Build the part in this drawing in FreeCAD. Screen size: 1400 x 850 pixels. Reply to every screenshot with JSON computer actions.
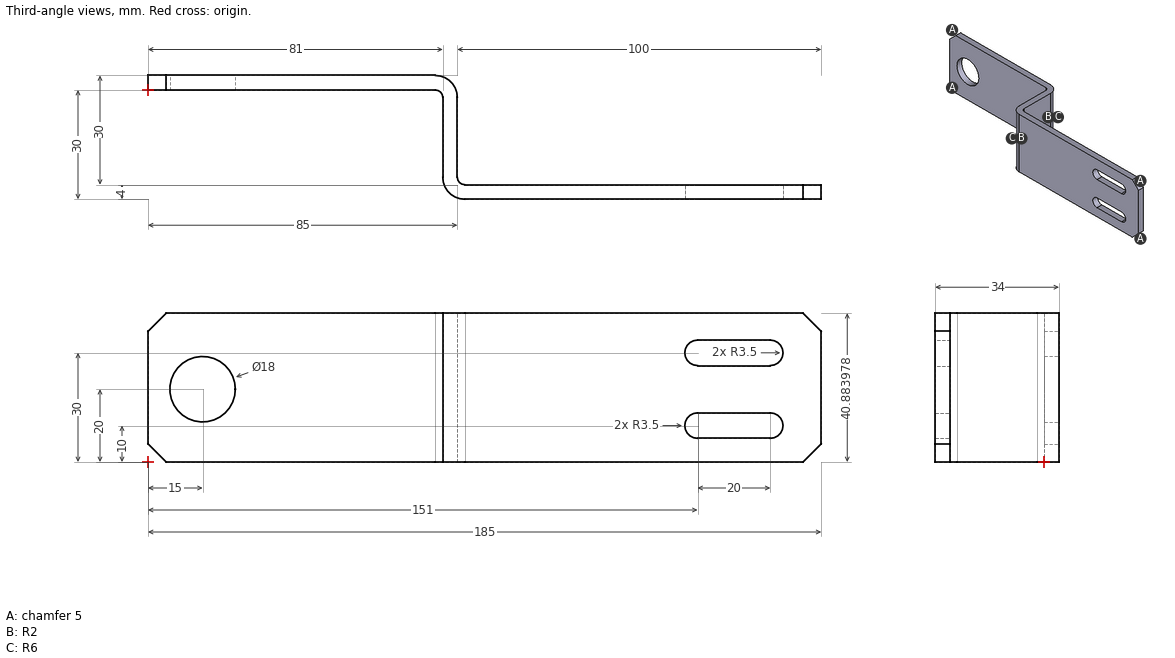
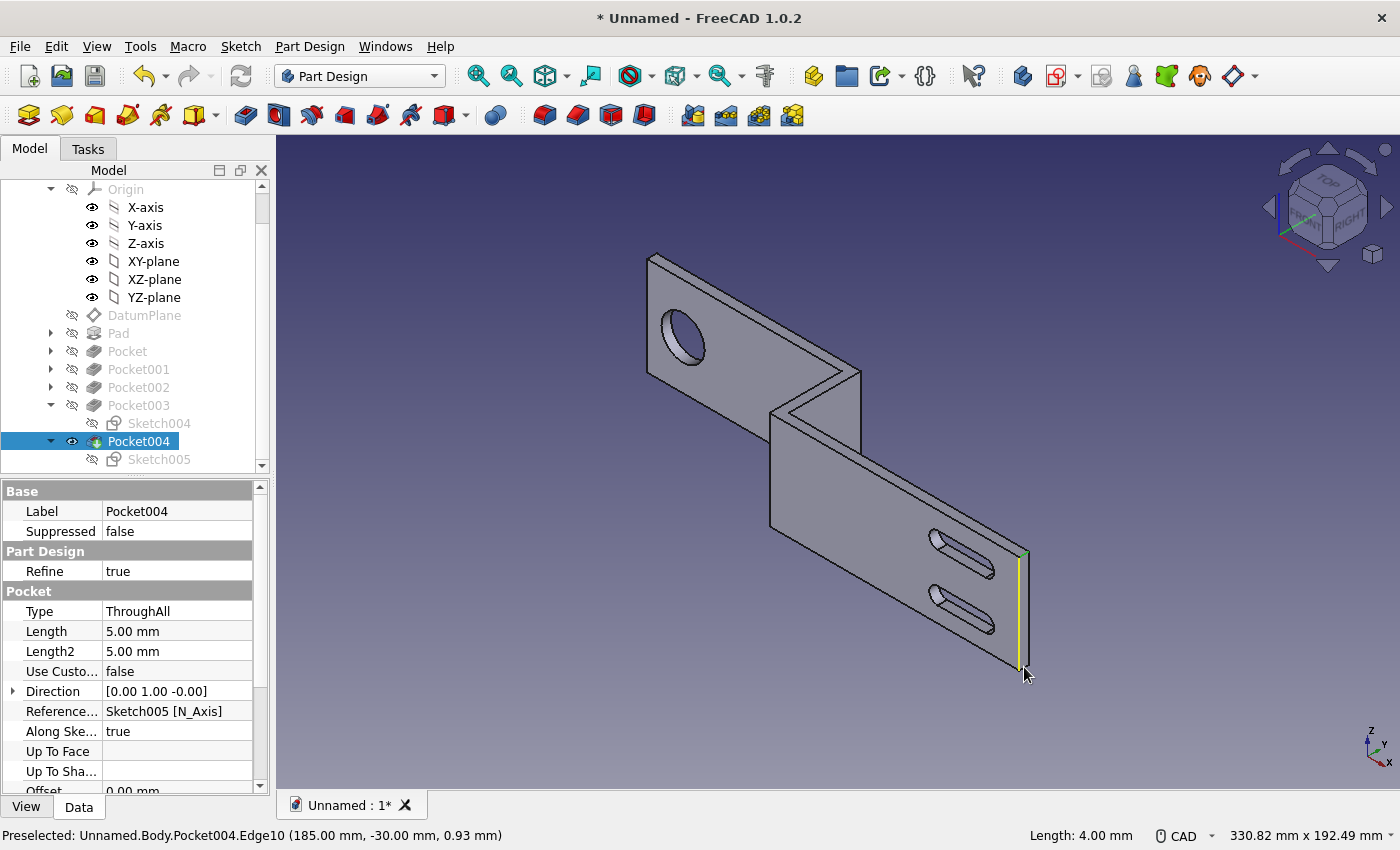
{"action": "key", "text": "2"}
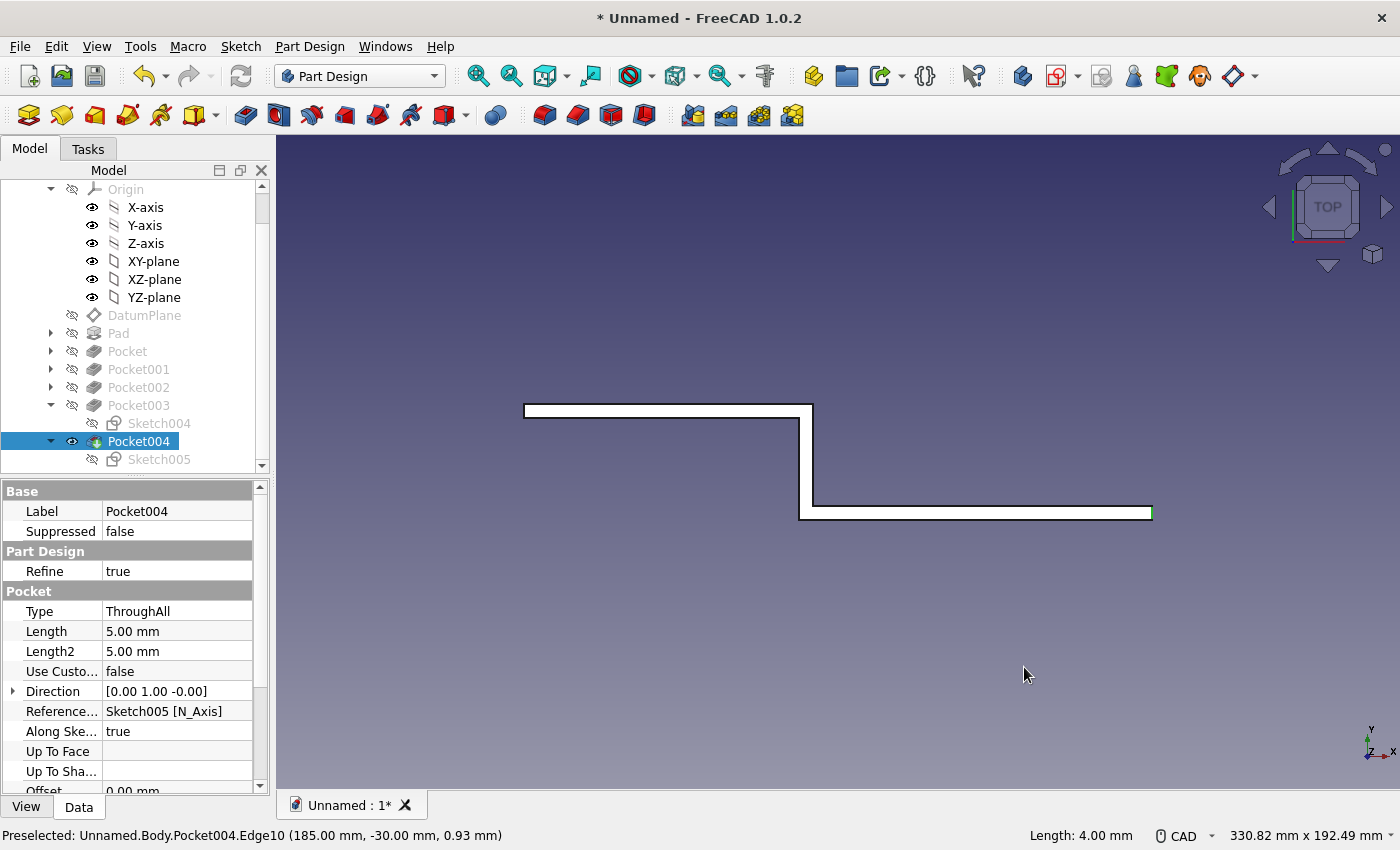
{"action": "left_click", "coordinate": [524, 410], "text": "ctrl"}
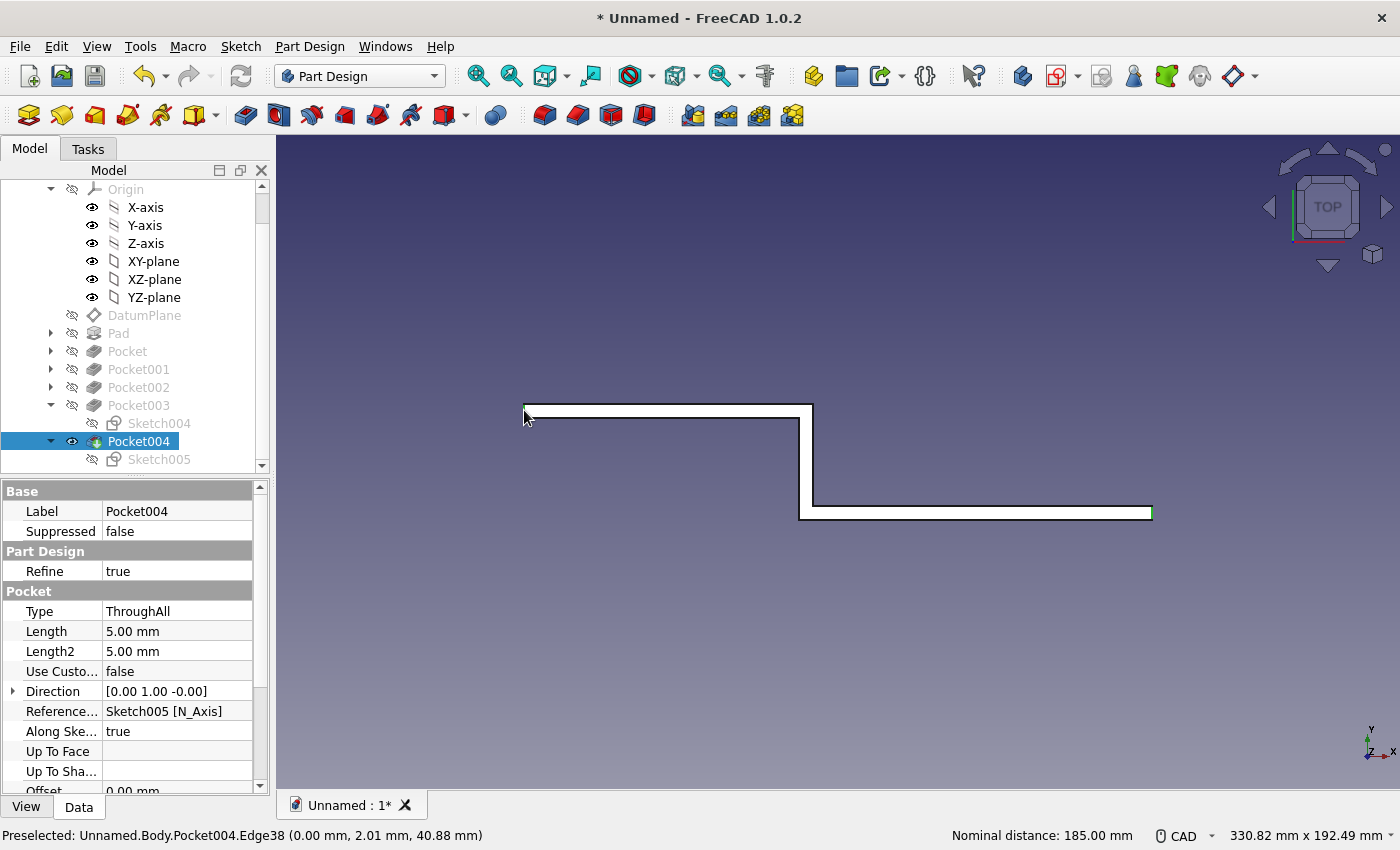
{"action": "scroll", "coordinate": [1152, 512], "scroll_direction": "up", "scroll_amount": 6}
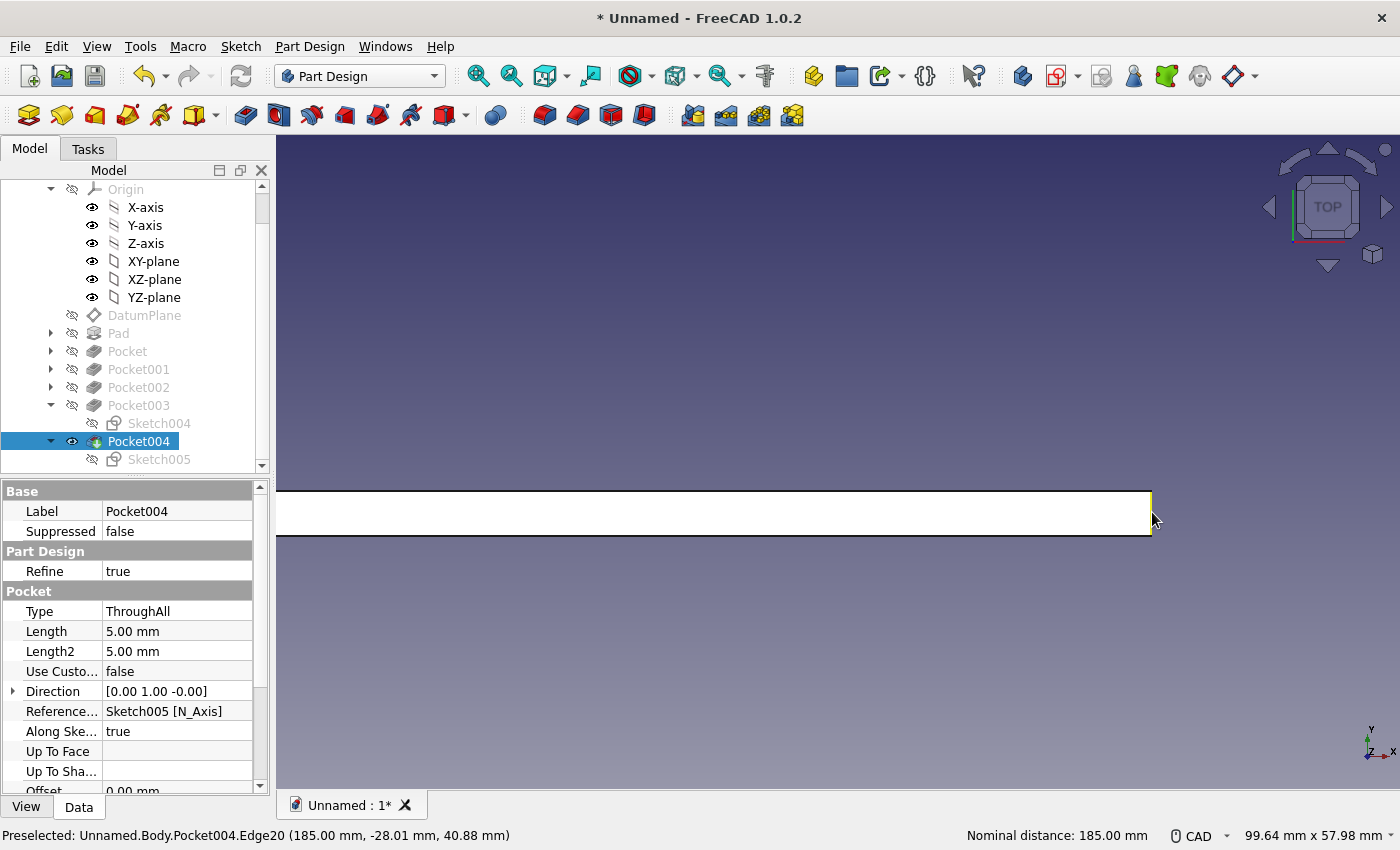
{"action": "left_click", "coordinate": [479, 76]}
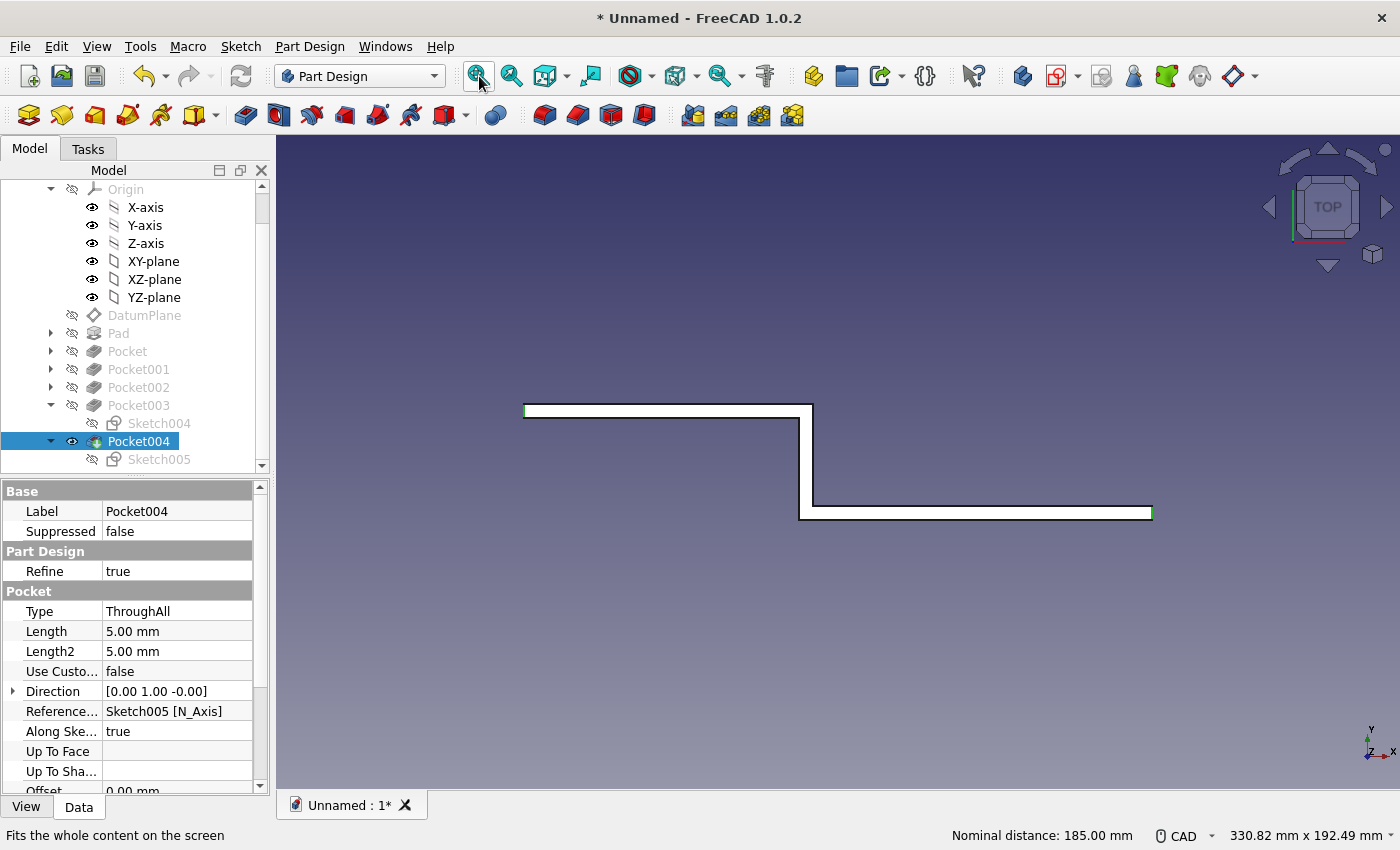
{"action": "key", "text": "0"}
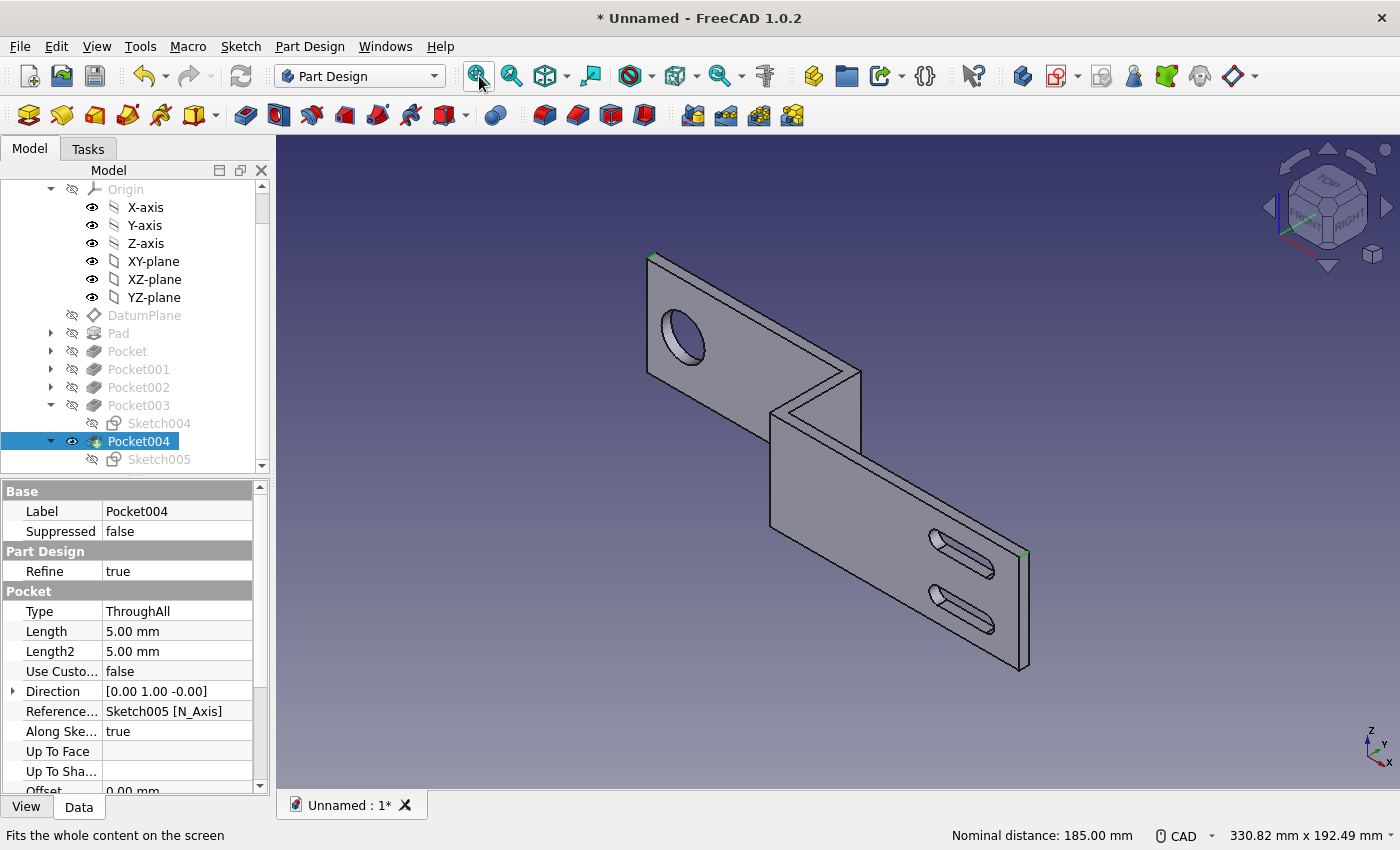
{"action": "scroll", "coordinate": [1024, 667], "scroll_direction": "up", "scroll_amount": 6}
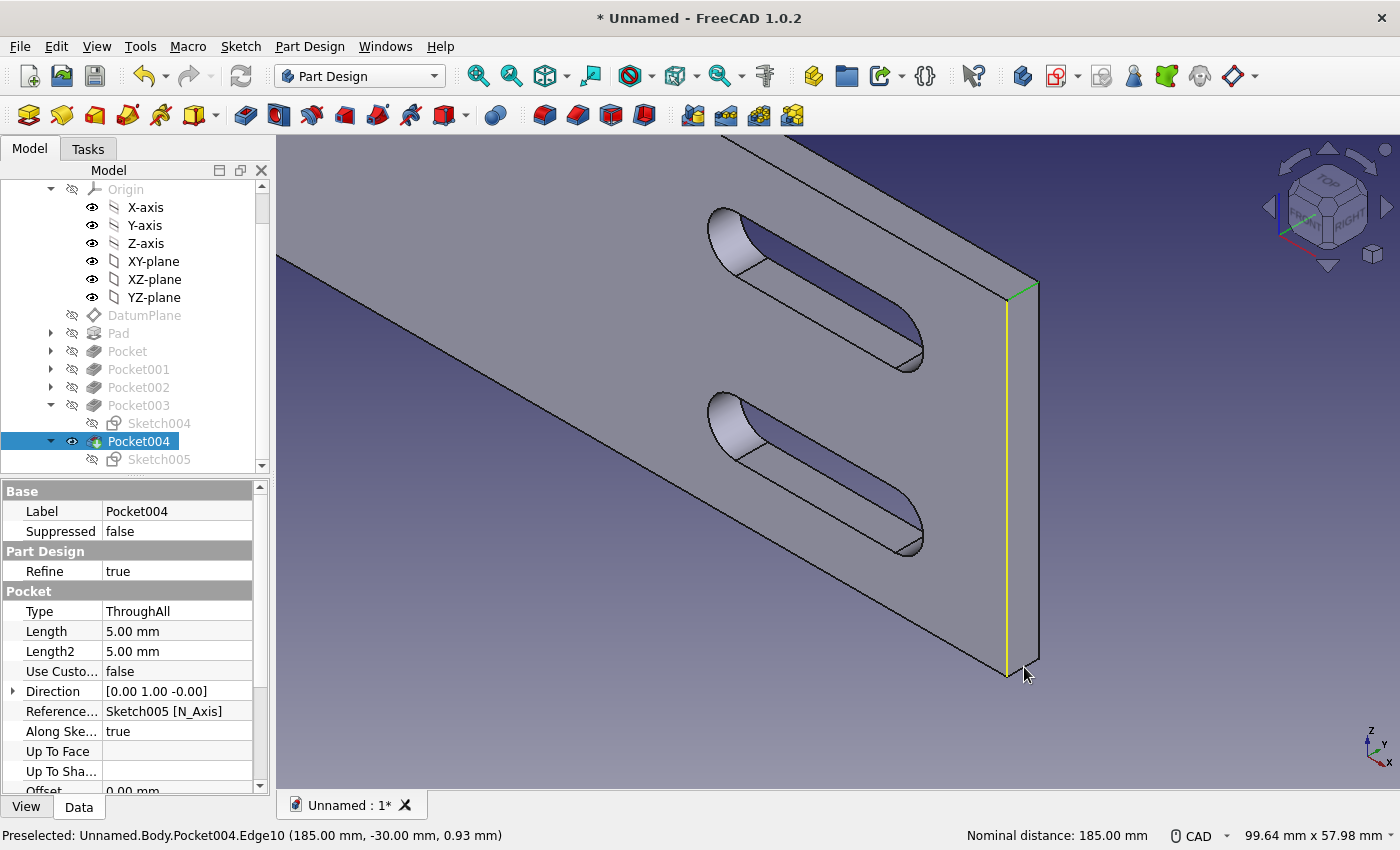
{"action": "key", "text": "v f"}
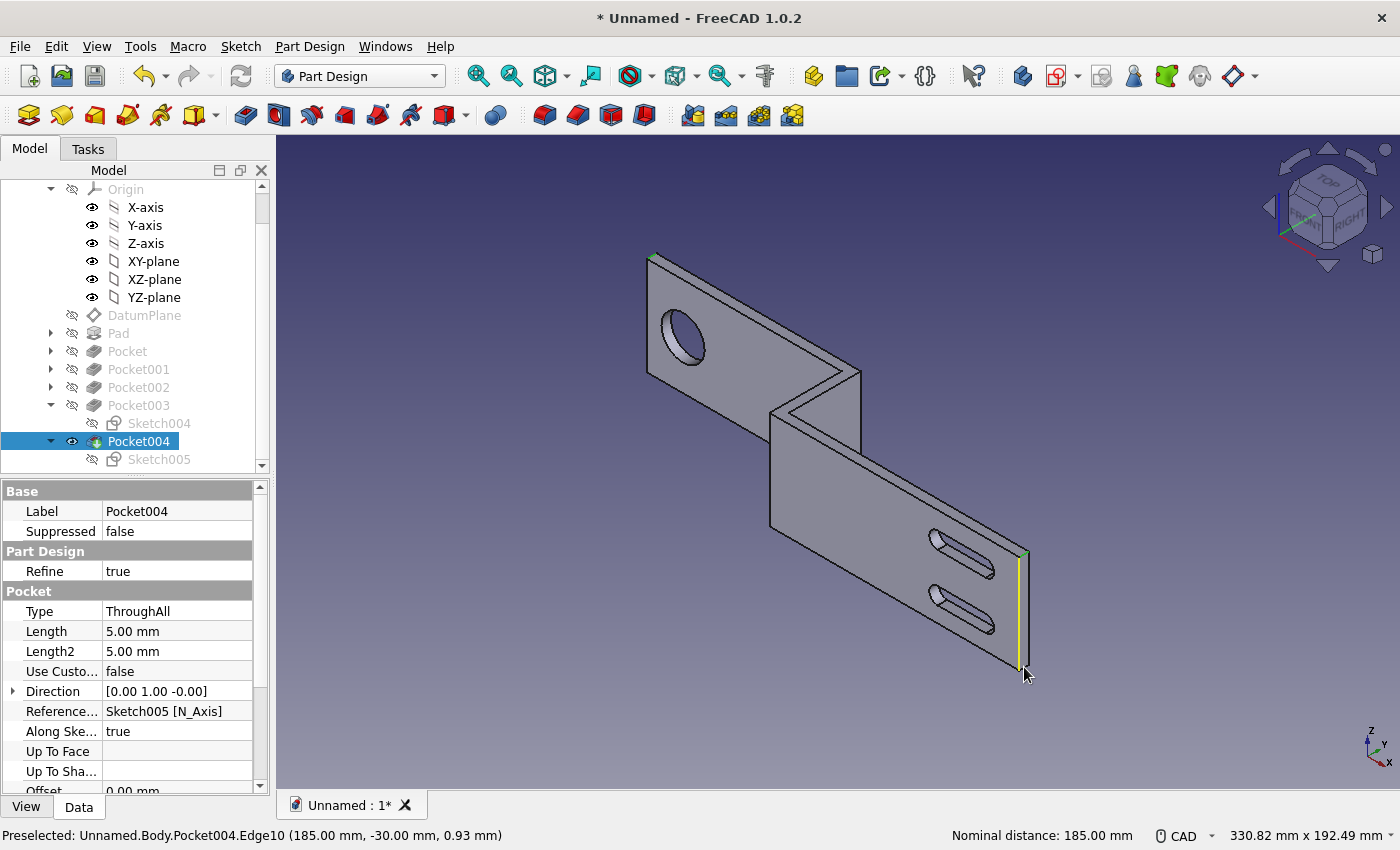
{"action": "key", "text": "1"}